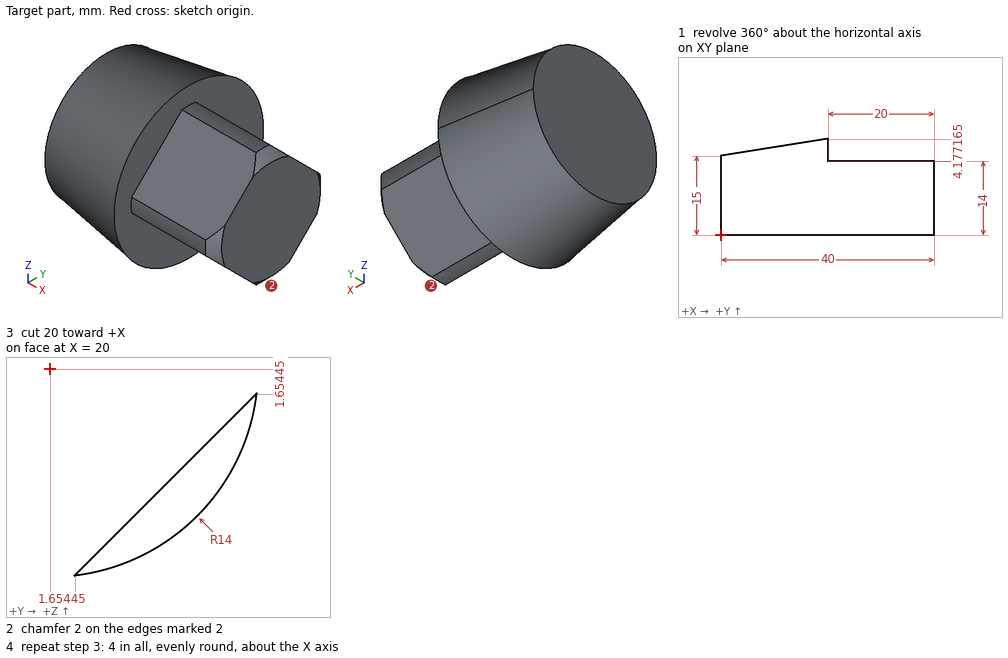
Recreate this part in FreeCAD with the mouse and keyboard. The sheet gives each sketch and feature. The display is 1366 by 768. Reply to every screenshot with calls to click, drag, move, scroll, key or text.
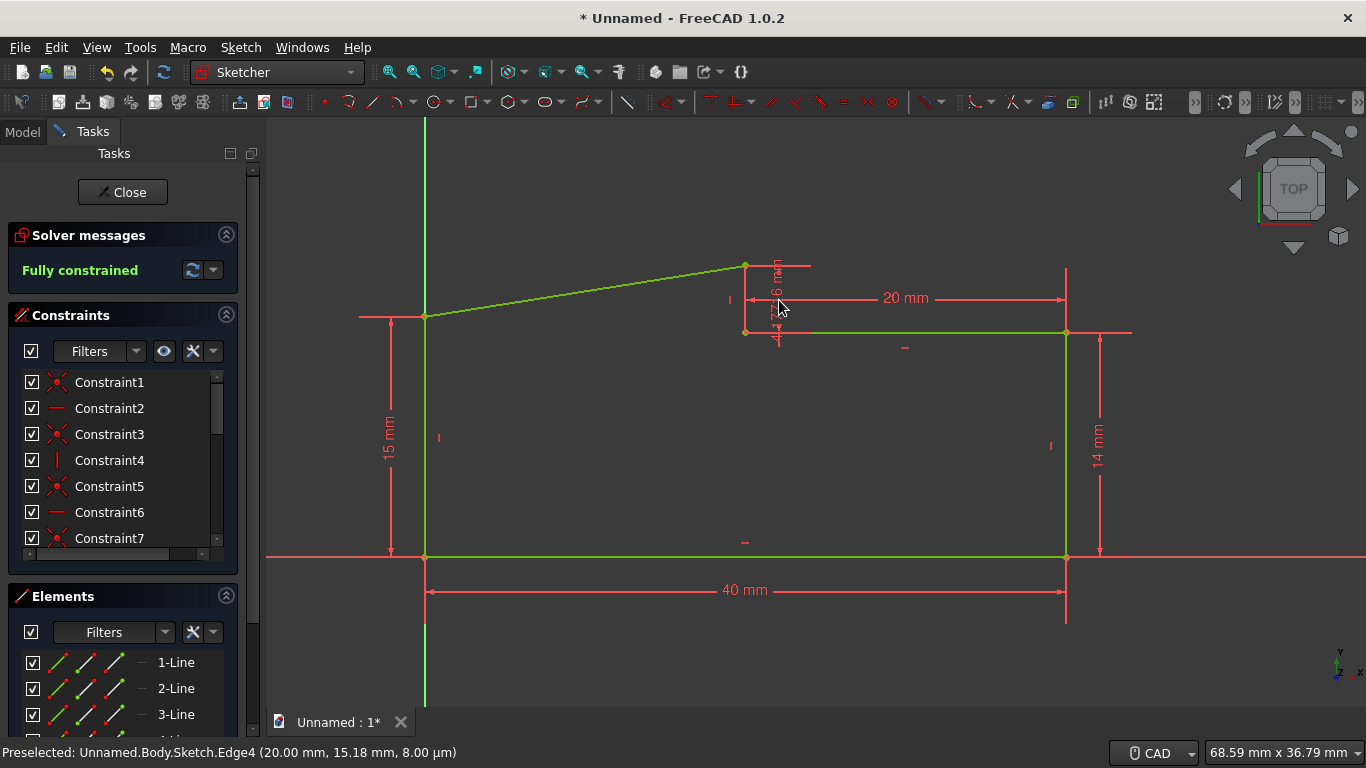
click(123, 192)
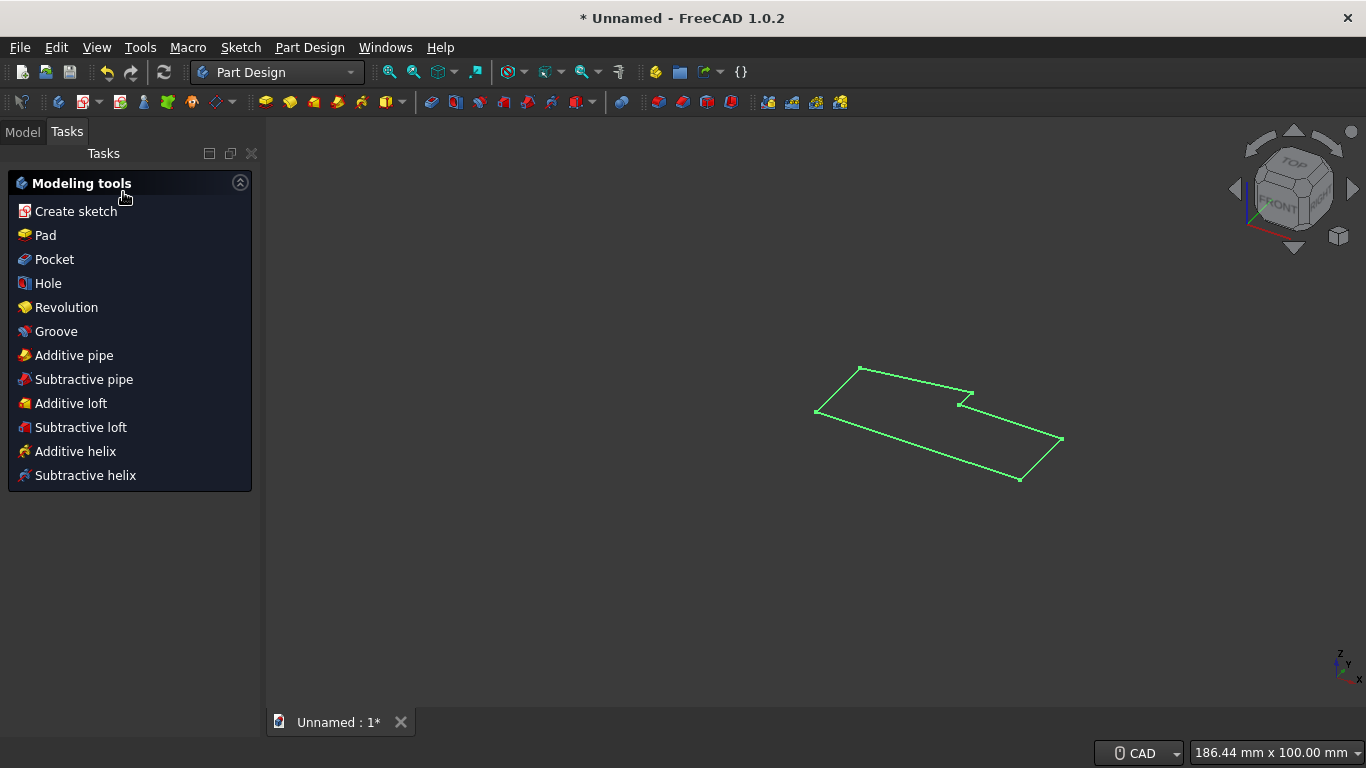
click(290, 102)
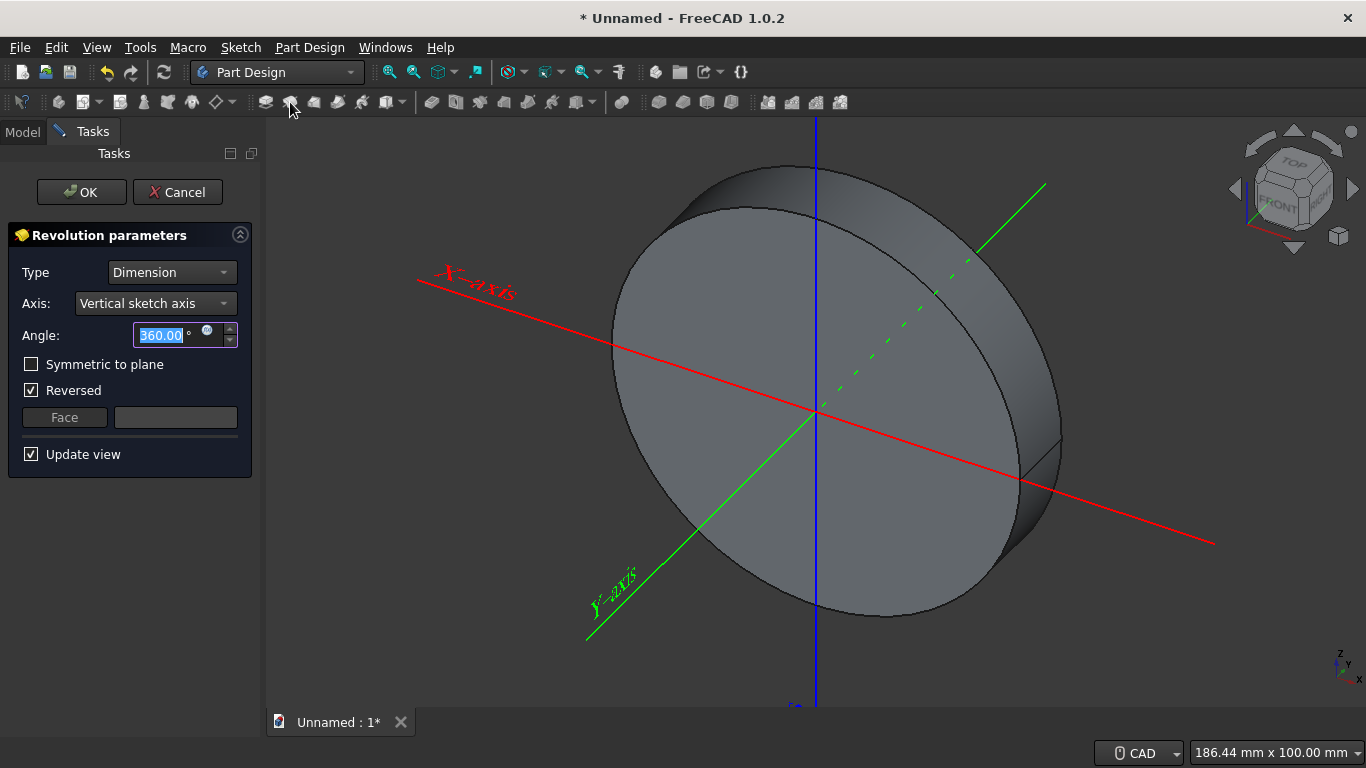
click(156, 304)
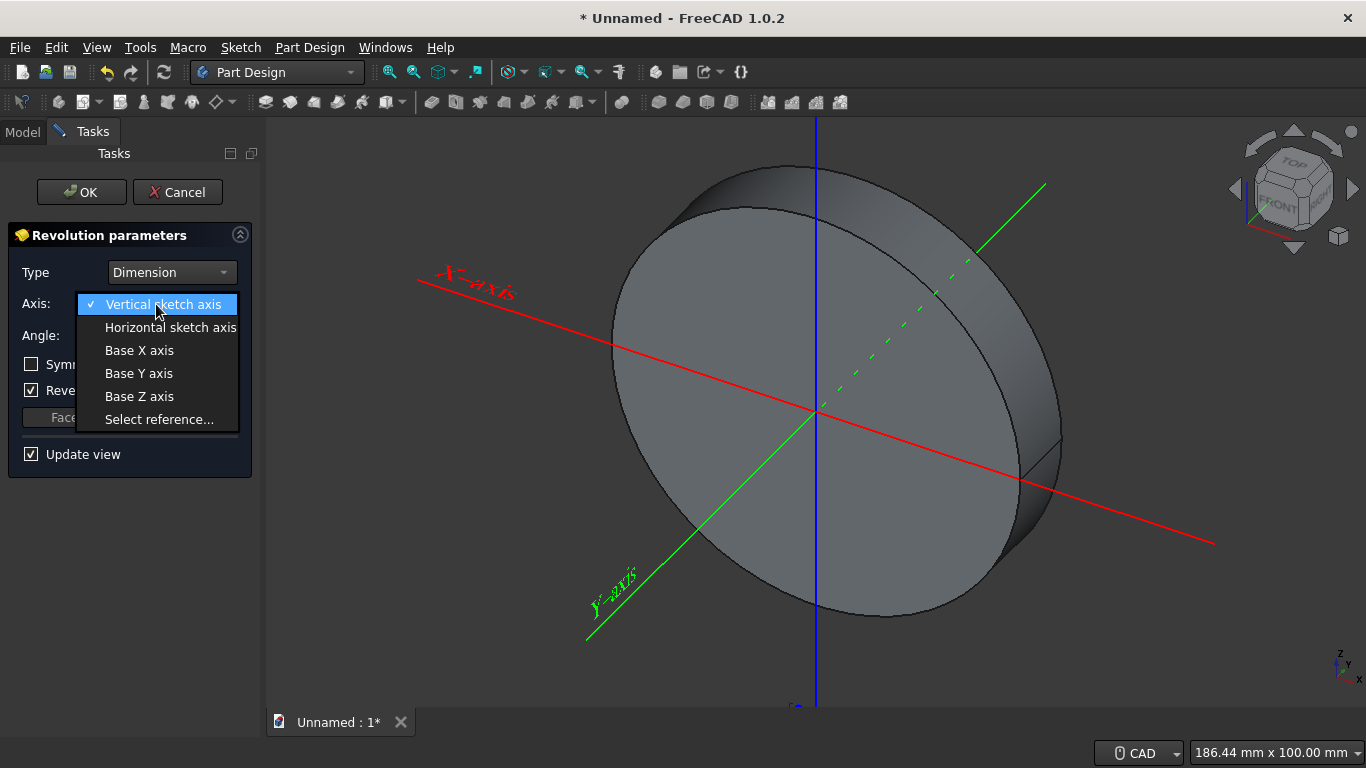
click(156, 328)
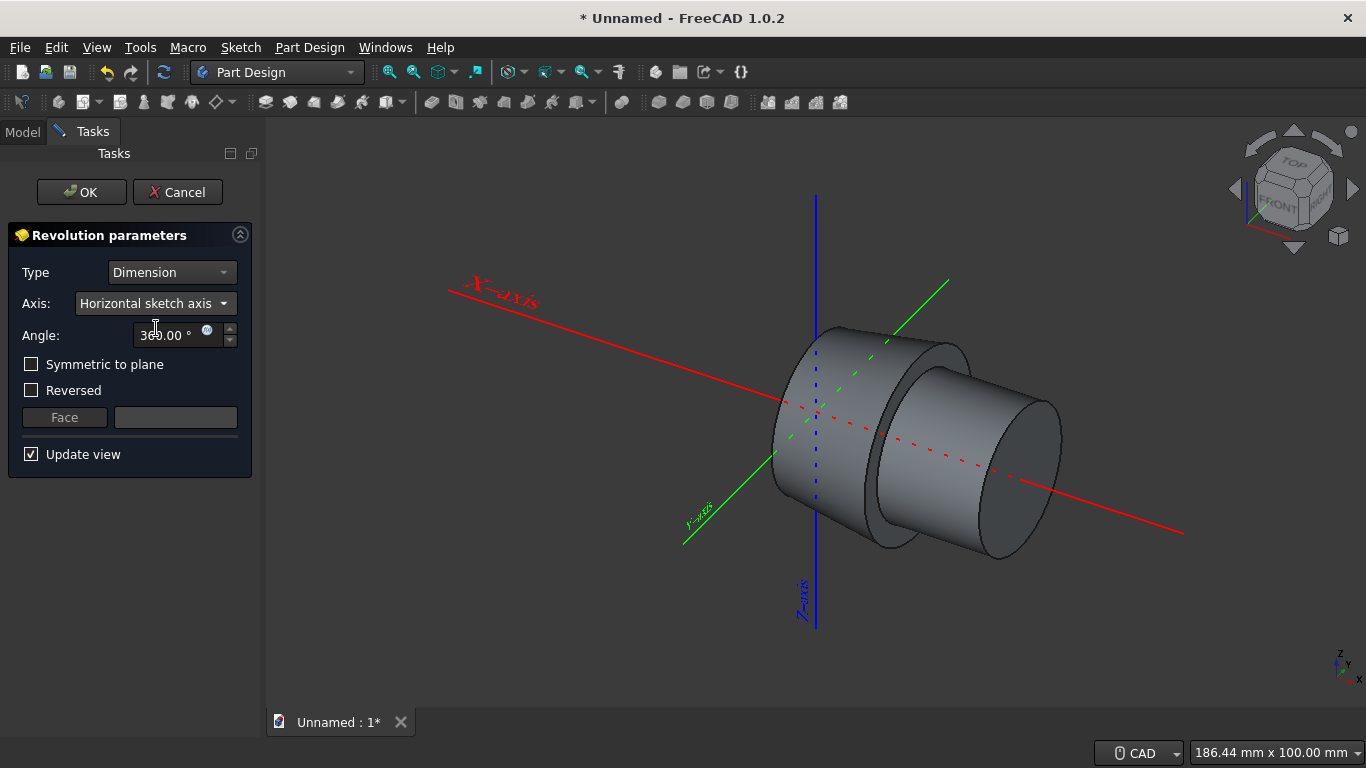
click(82, 192)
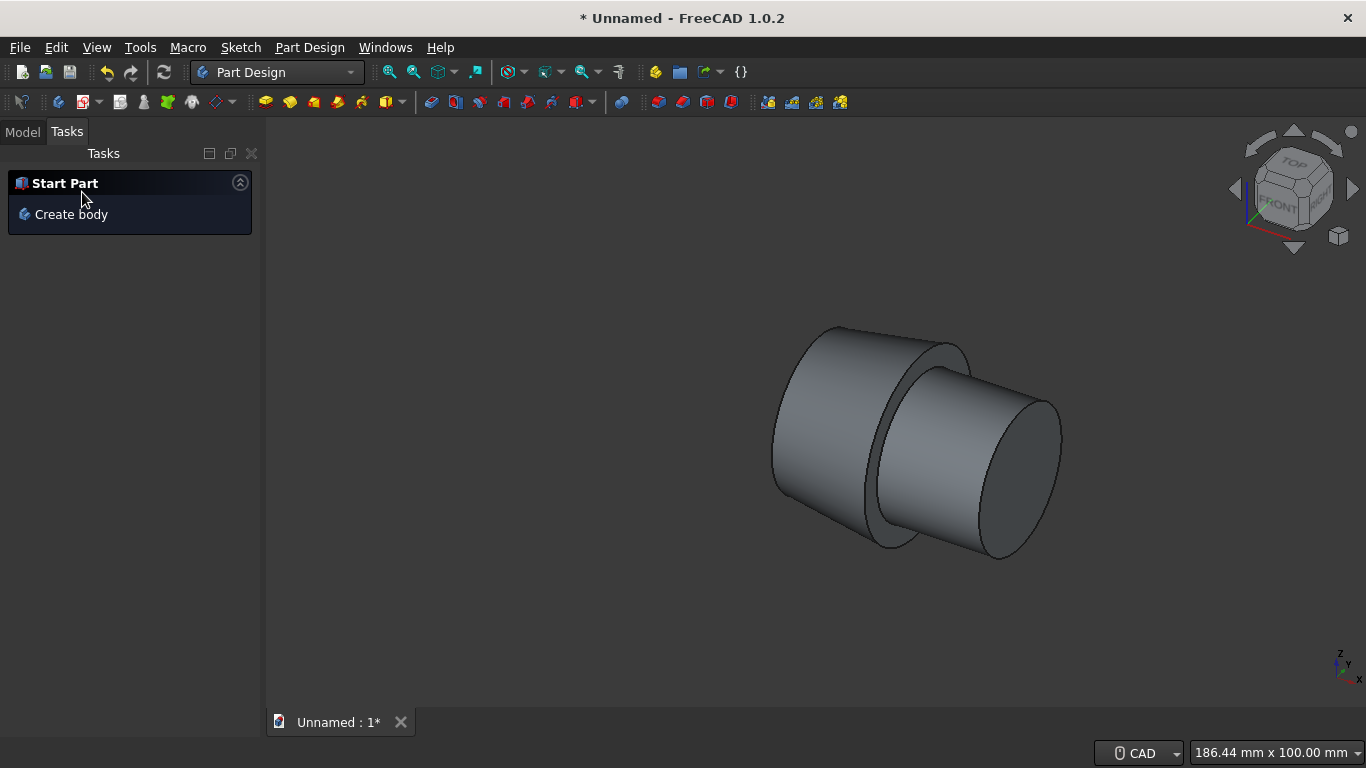
click(979, 520)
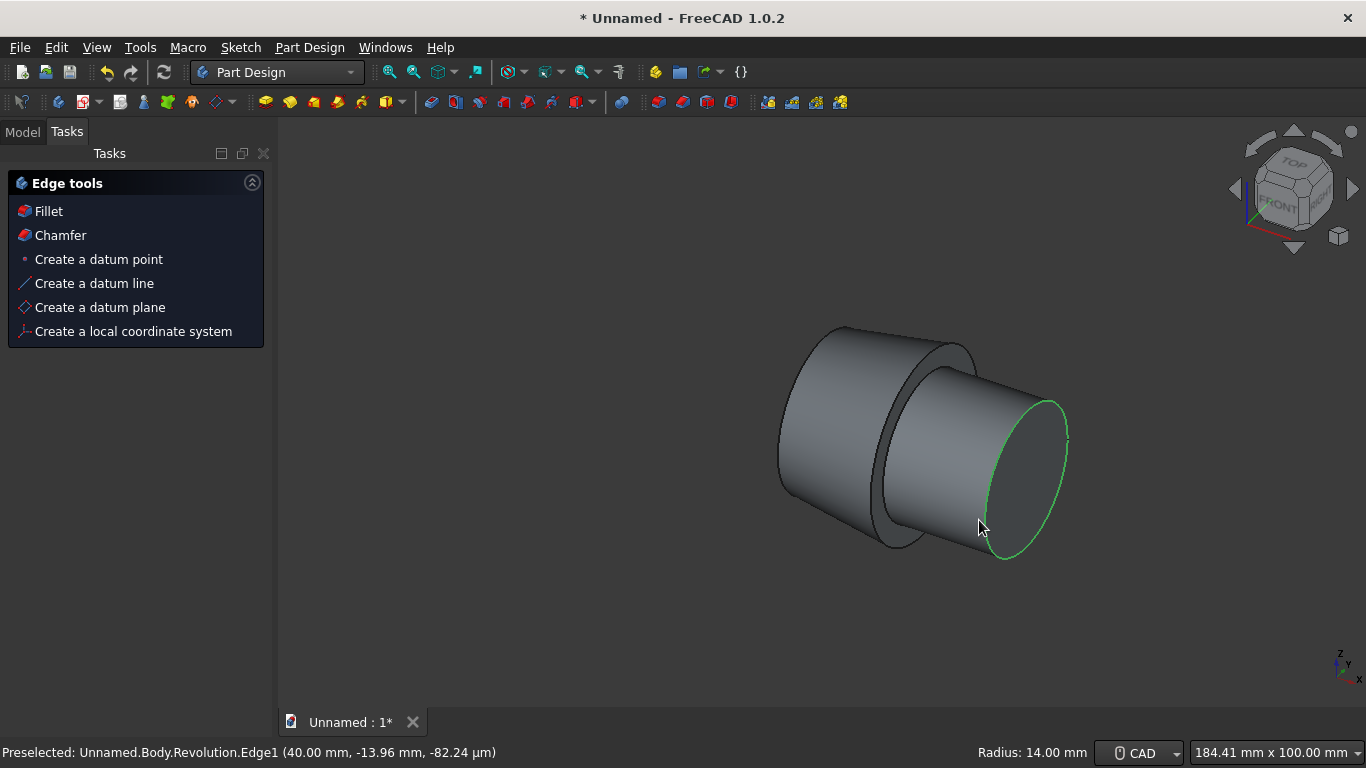
click(684, 102)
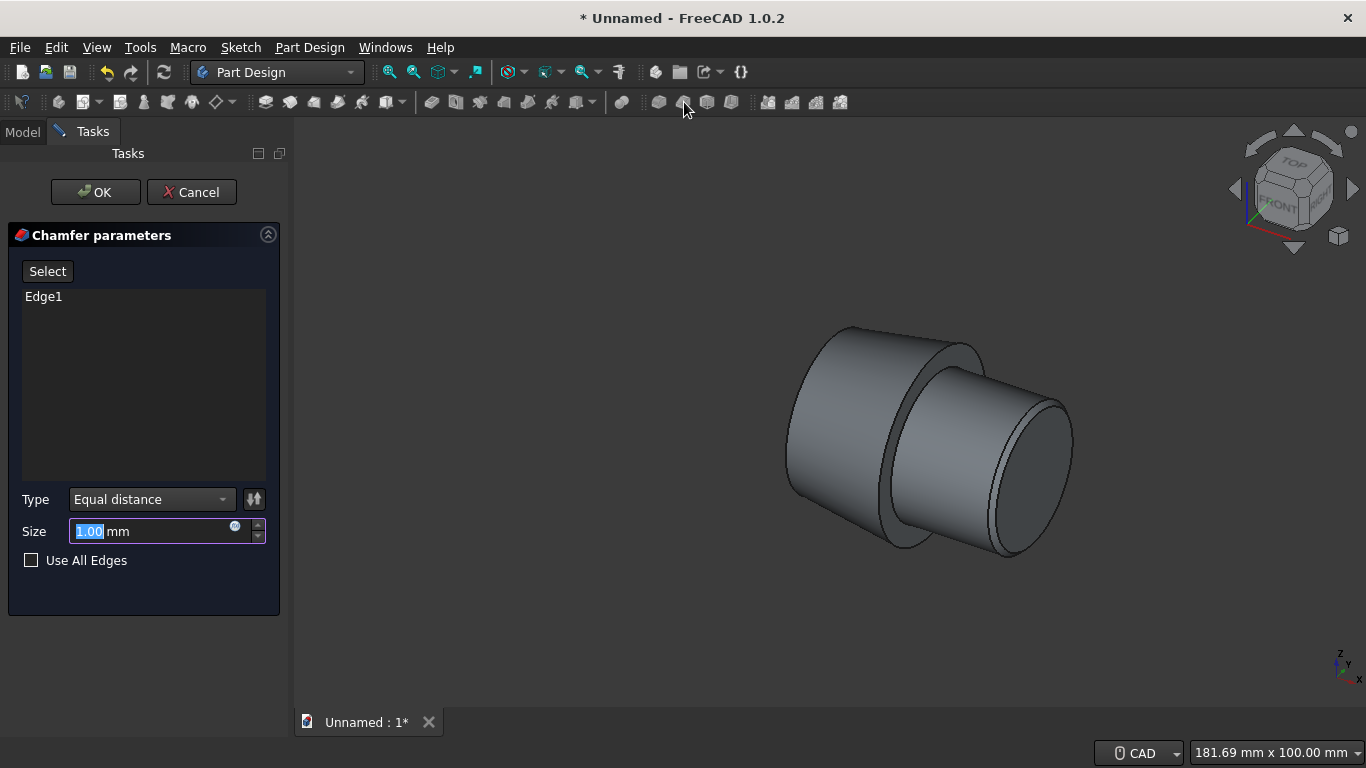
text(2)
key(Tab)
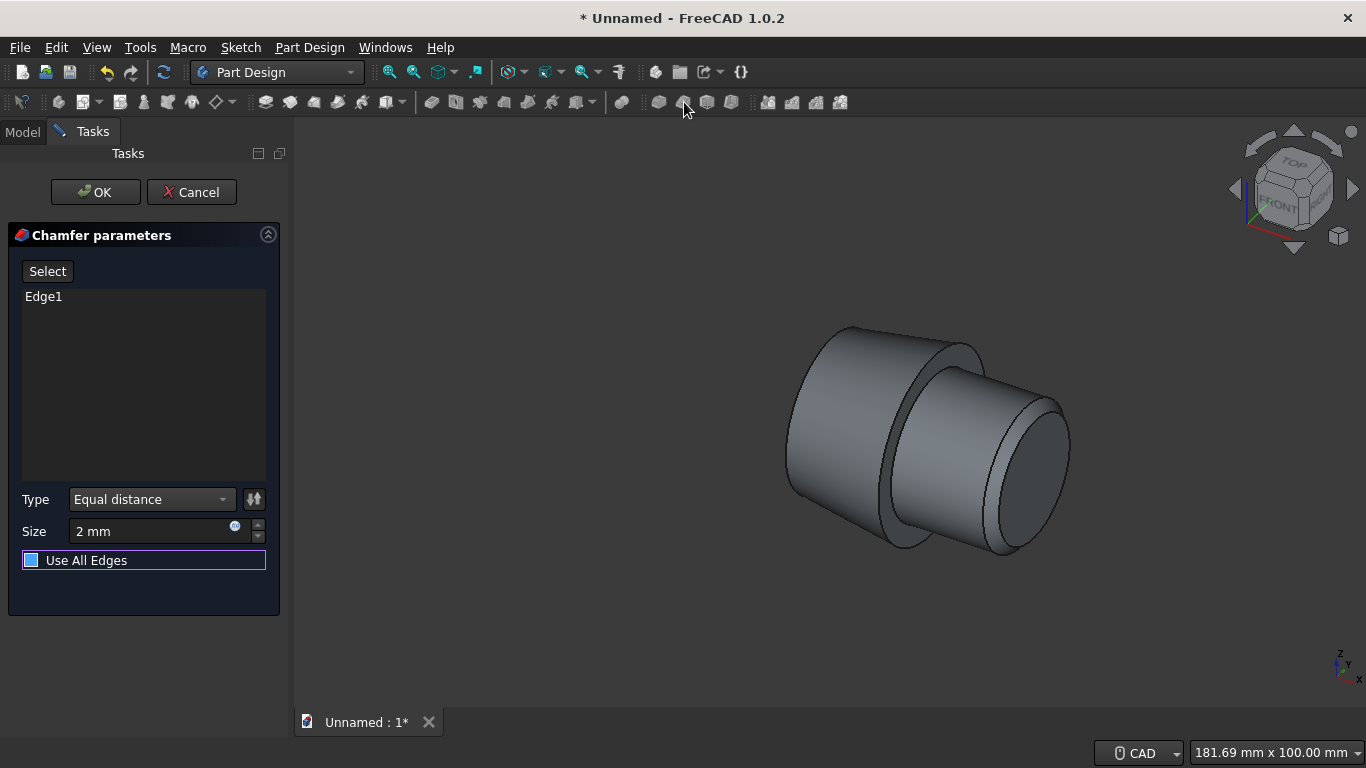
click(96, 192)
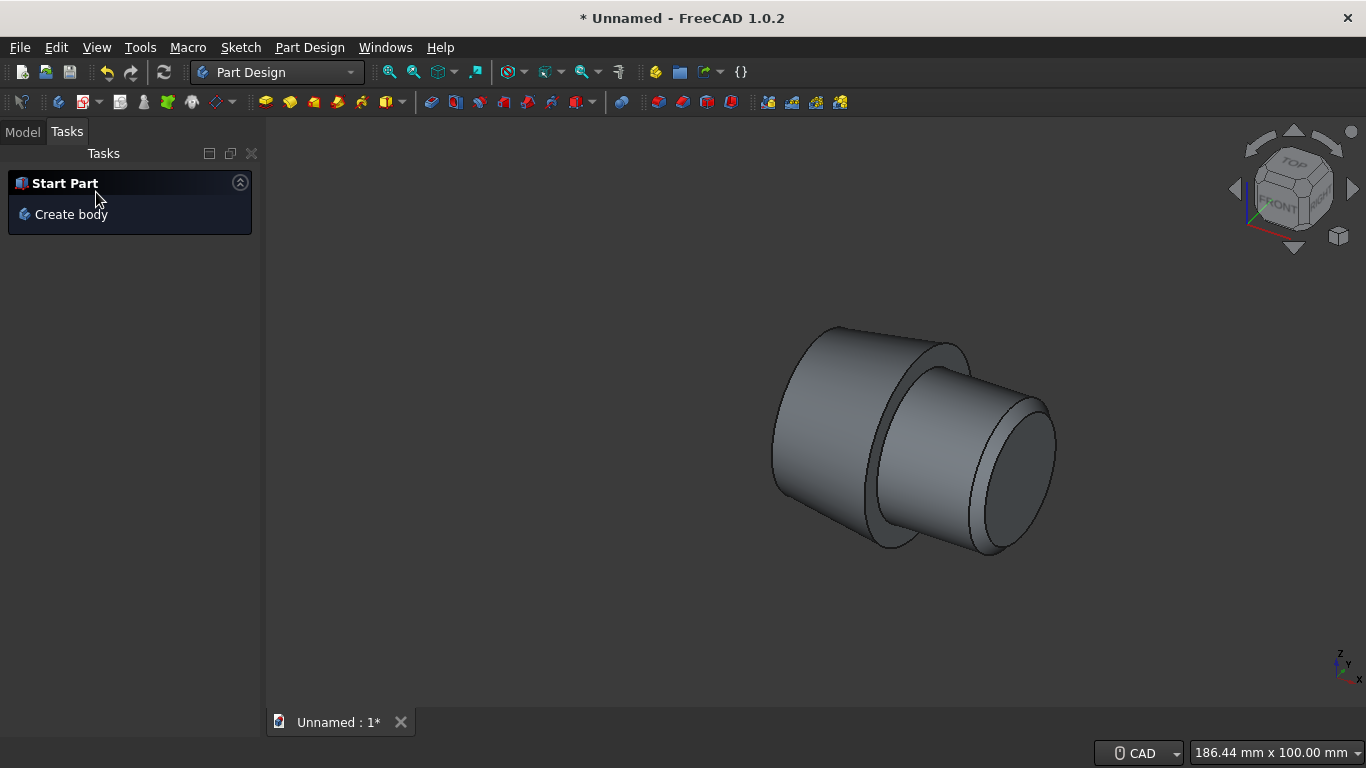
click(903, 535)